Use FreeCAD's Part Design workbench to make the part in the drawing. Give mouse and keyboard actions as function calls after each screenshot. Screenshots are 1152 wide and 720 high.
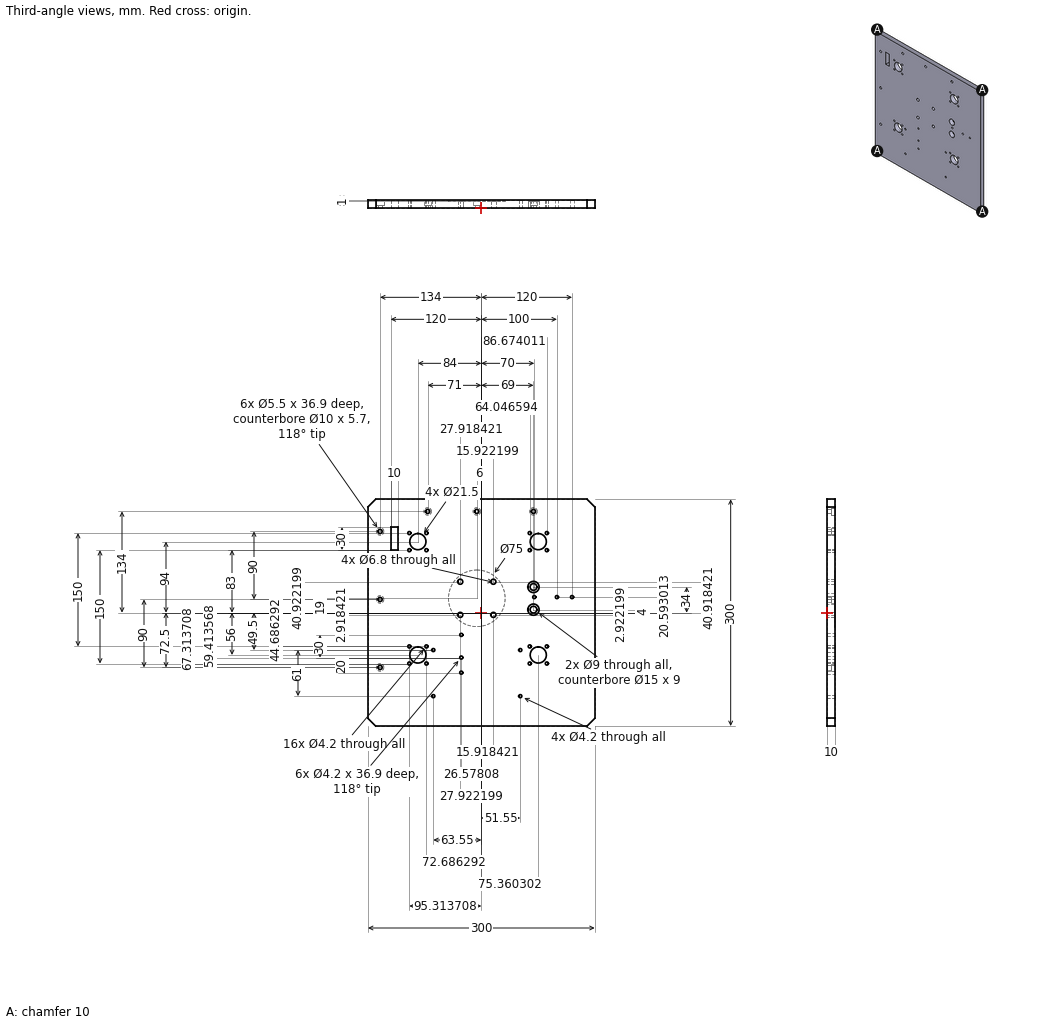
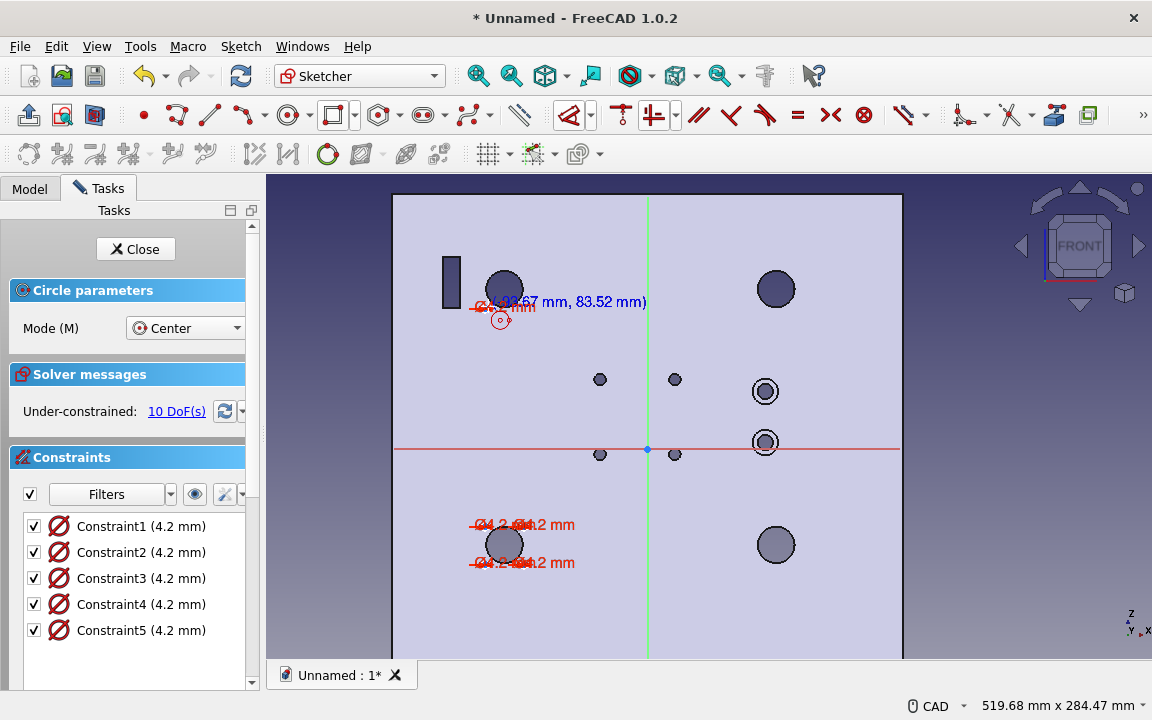
scroll(485, 270, up, 10)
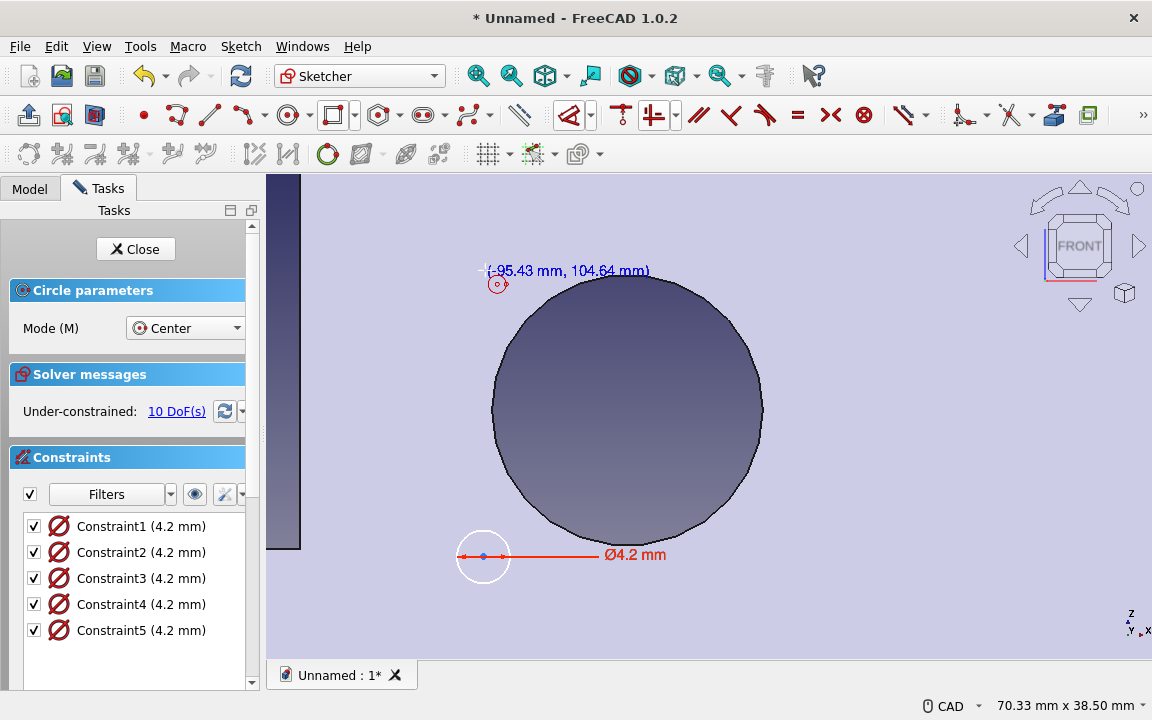
scroll(485, 270, down, 10)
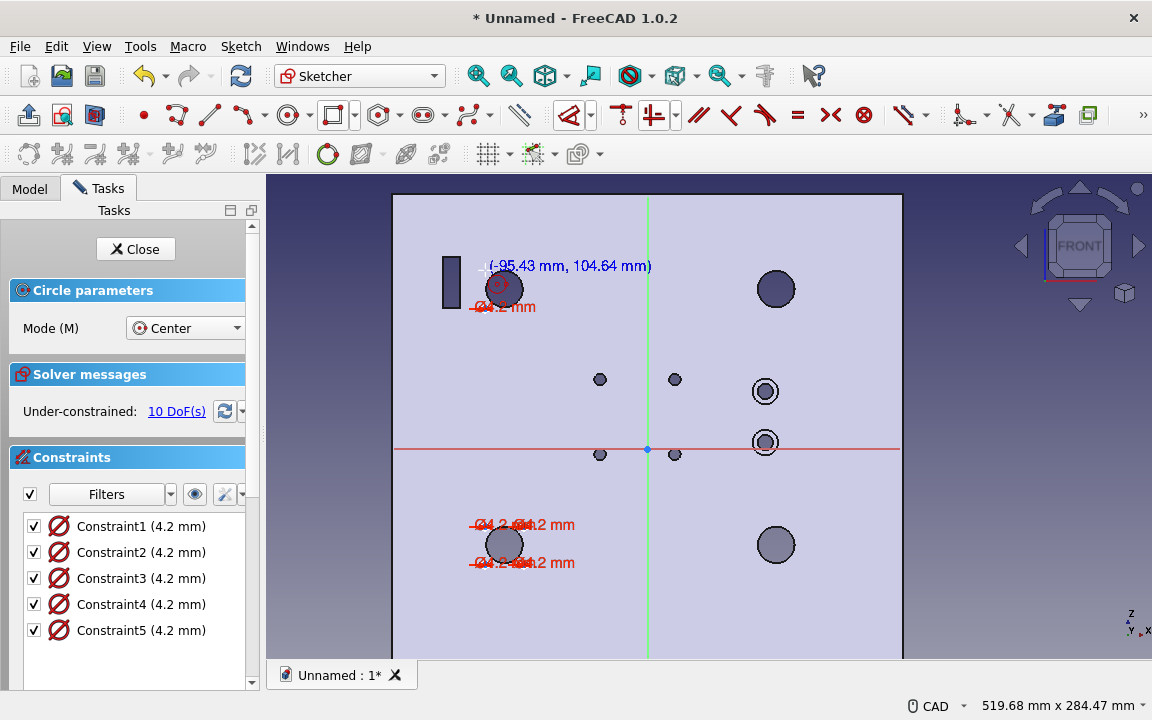
click(485, 270)
move(488, 267)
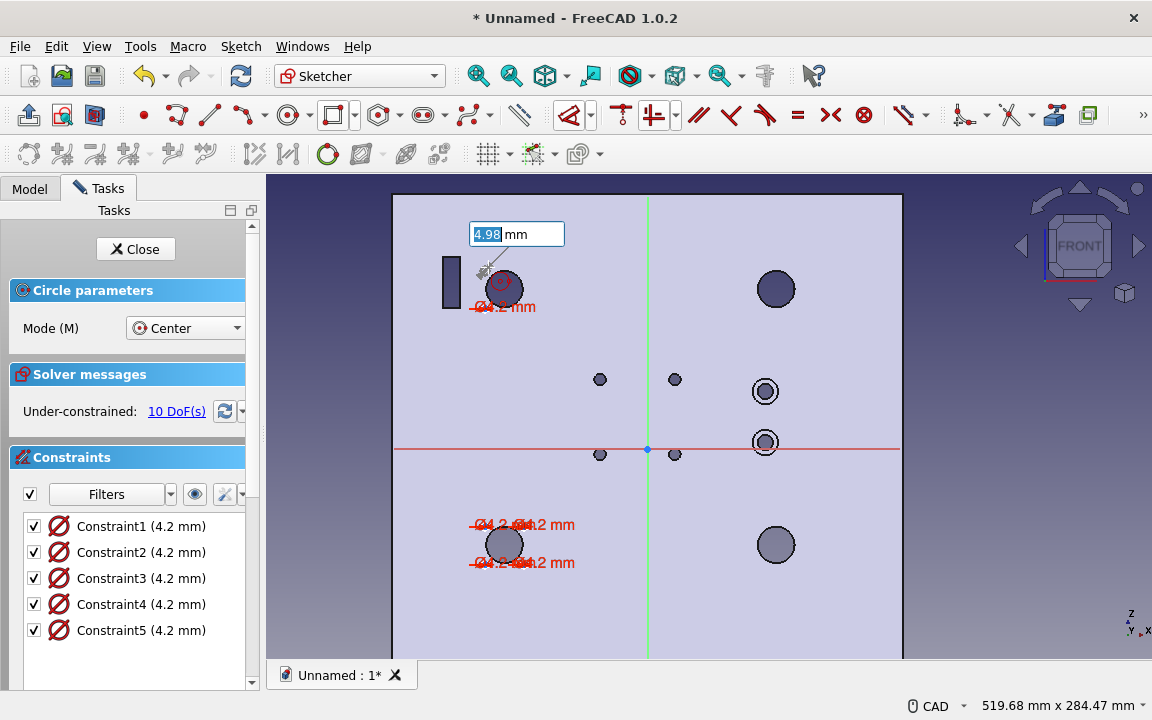
text(4.2)
key(Return)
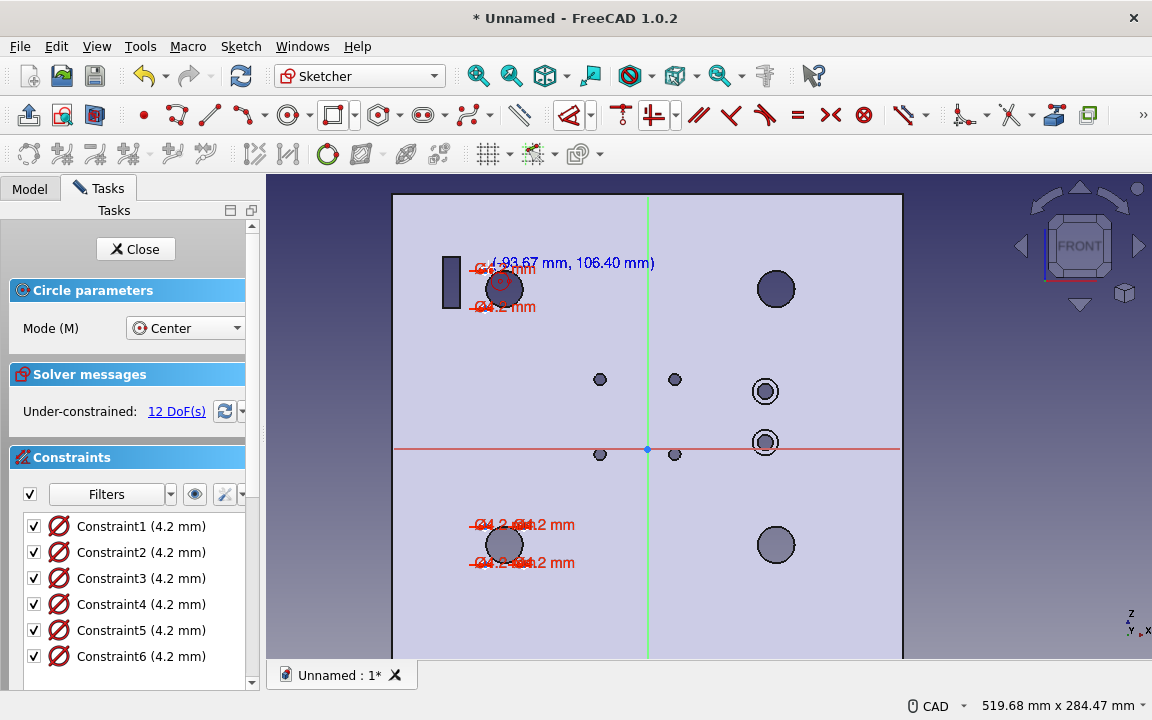
scroll(524, 270, up, 10)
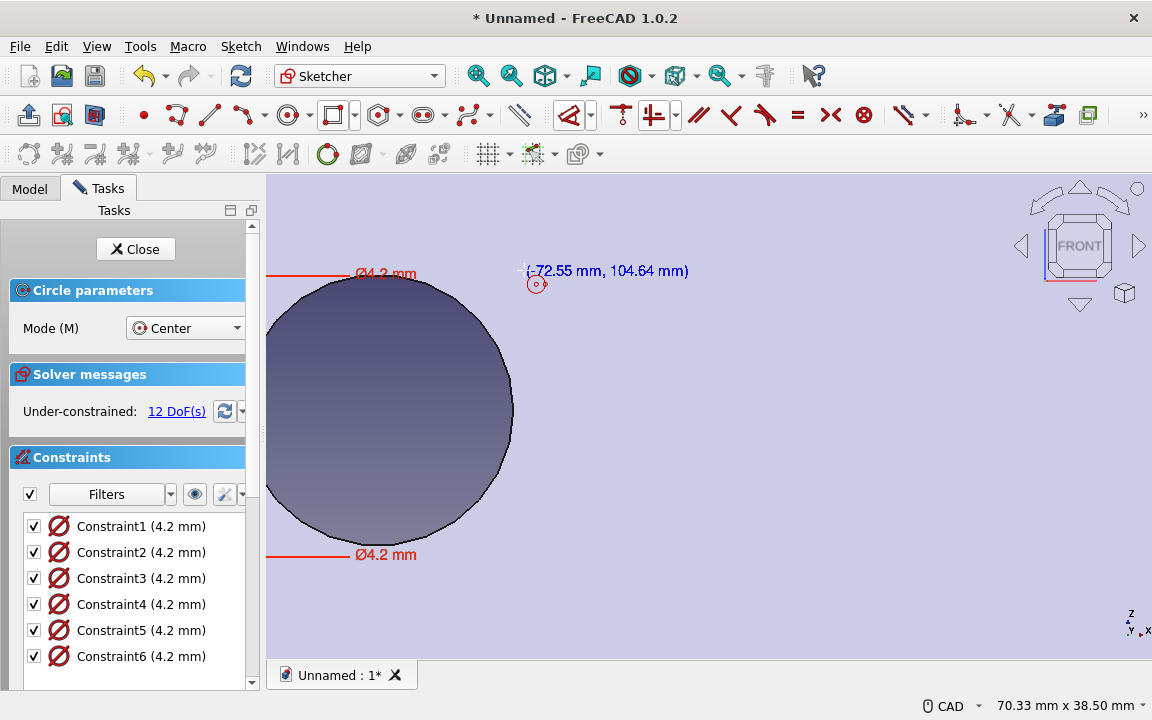
scroll(524, 270, down, 10)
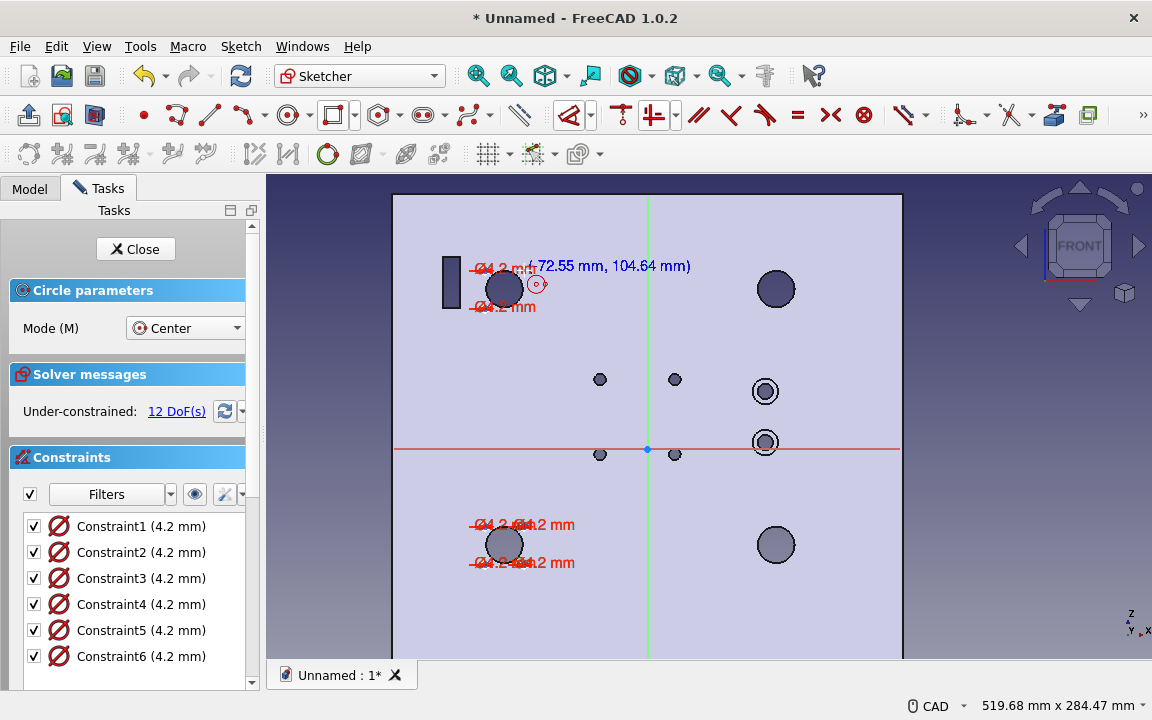
click(524, 270)
move(526, 267)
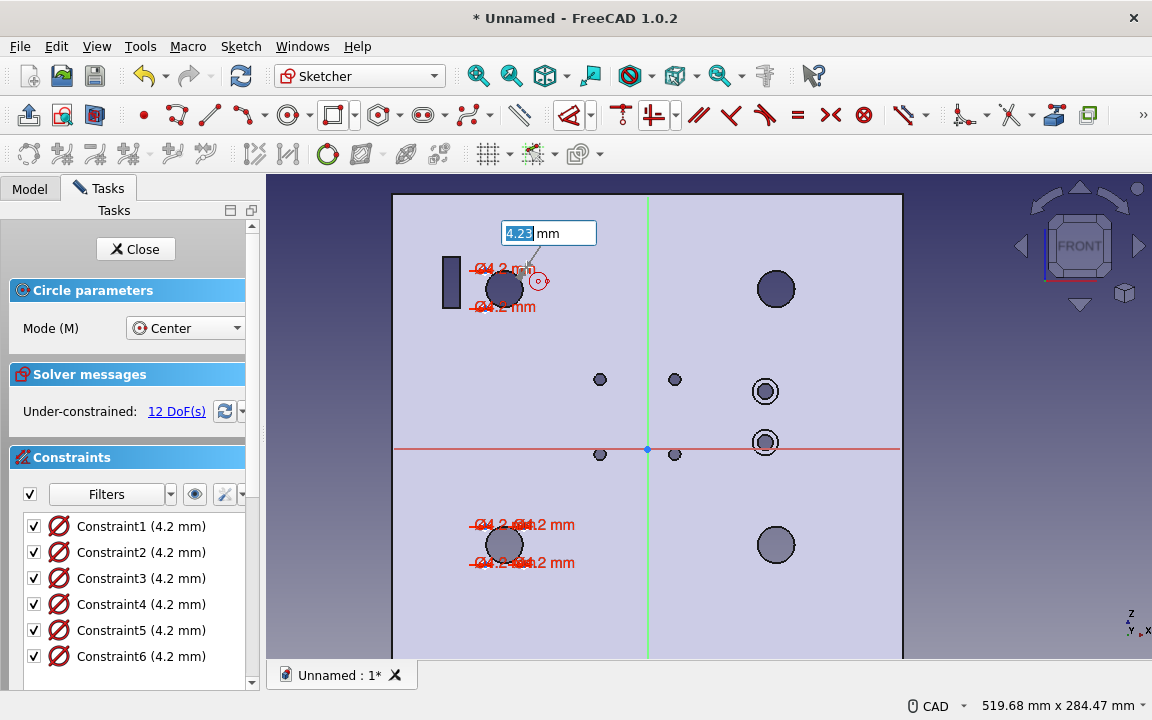
text(4.2)
key(Return)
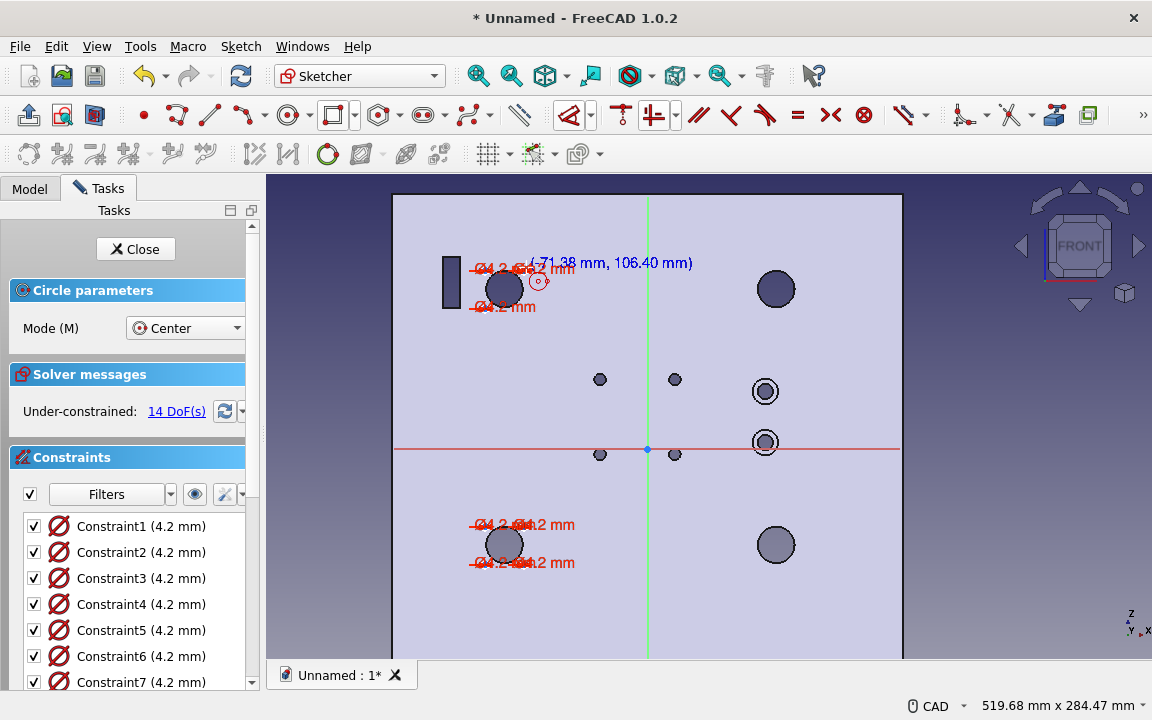
scroll(524, 308, up, 10)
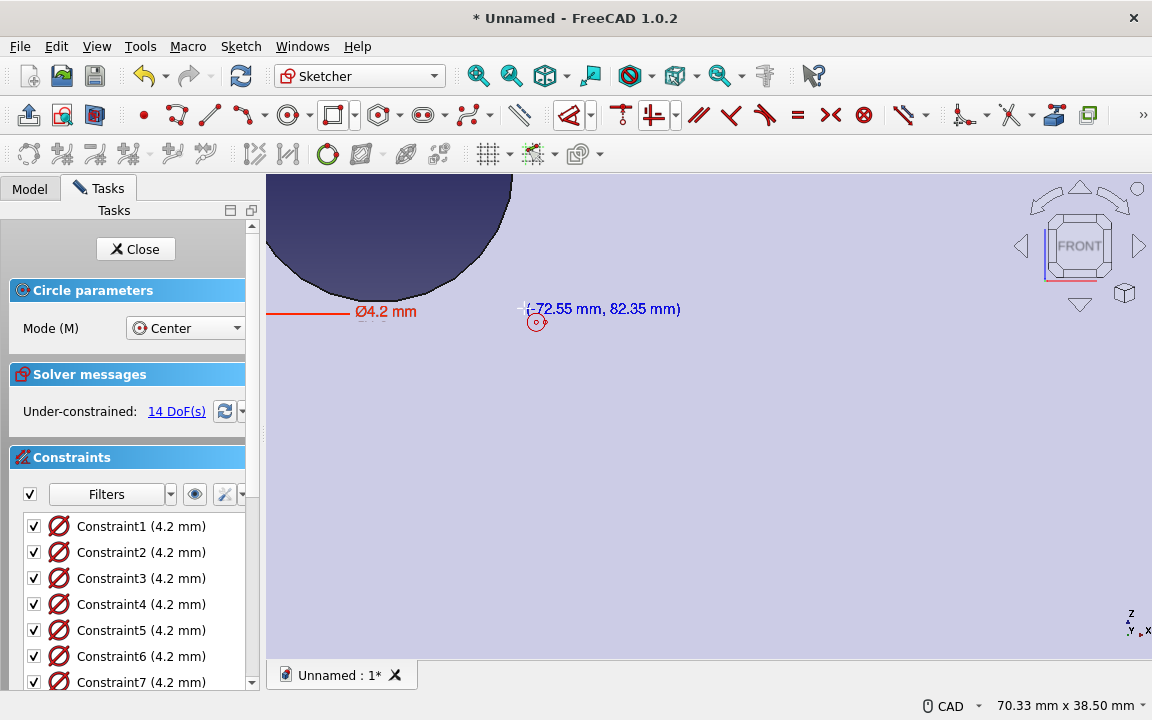
scroll(524, 308, down, 10)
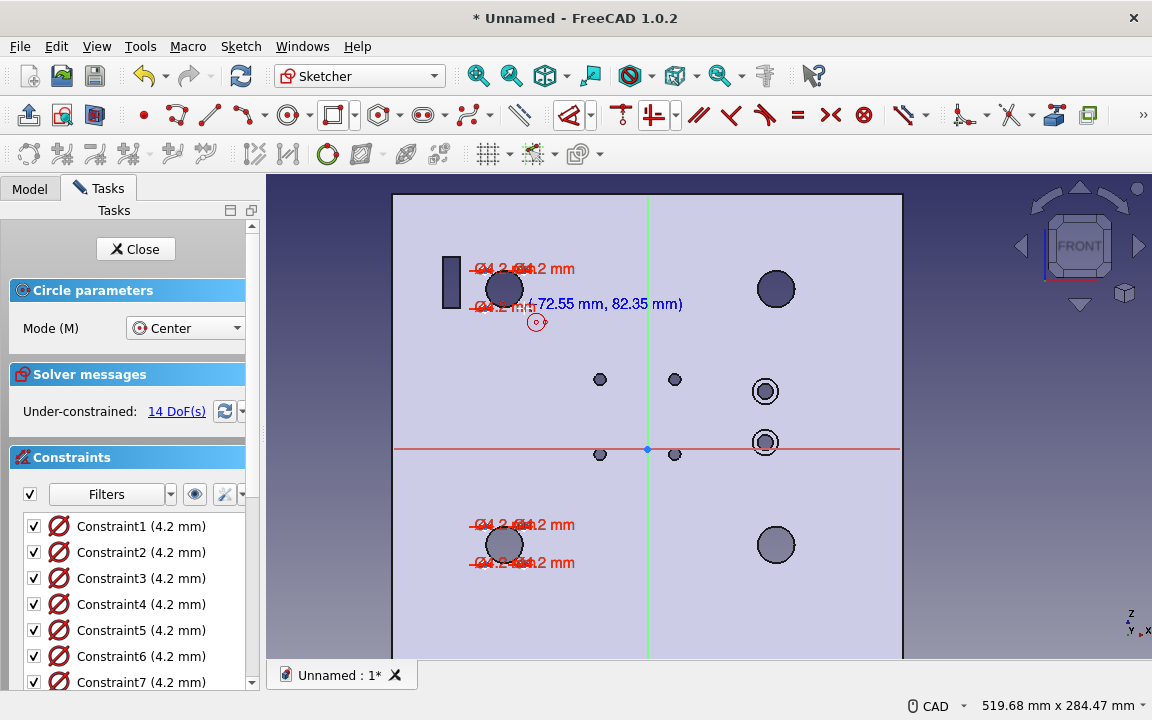
click(524, 308)
move(526, 306)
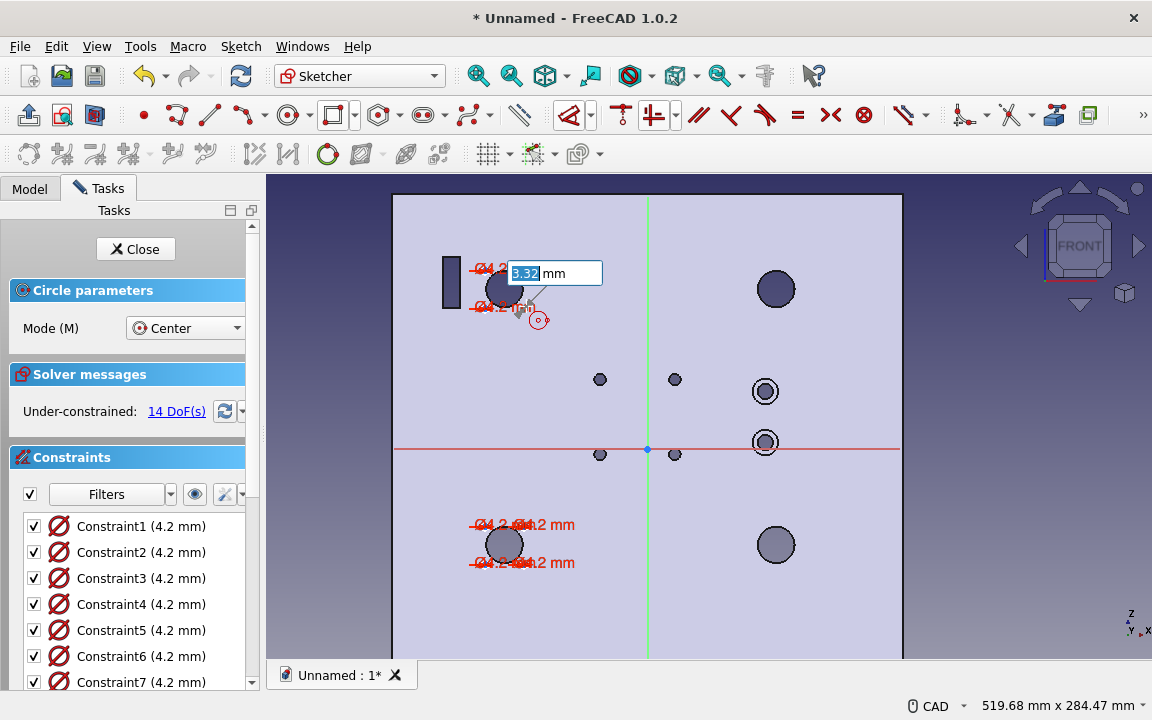
text(4.2)
key(Return)